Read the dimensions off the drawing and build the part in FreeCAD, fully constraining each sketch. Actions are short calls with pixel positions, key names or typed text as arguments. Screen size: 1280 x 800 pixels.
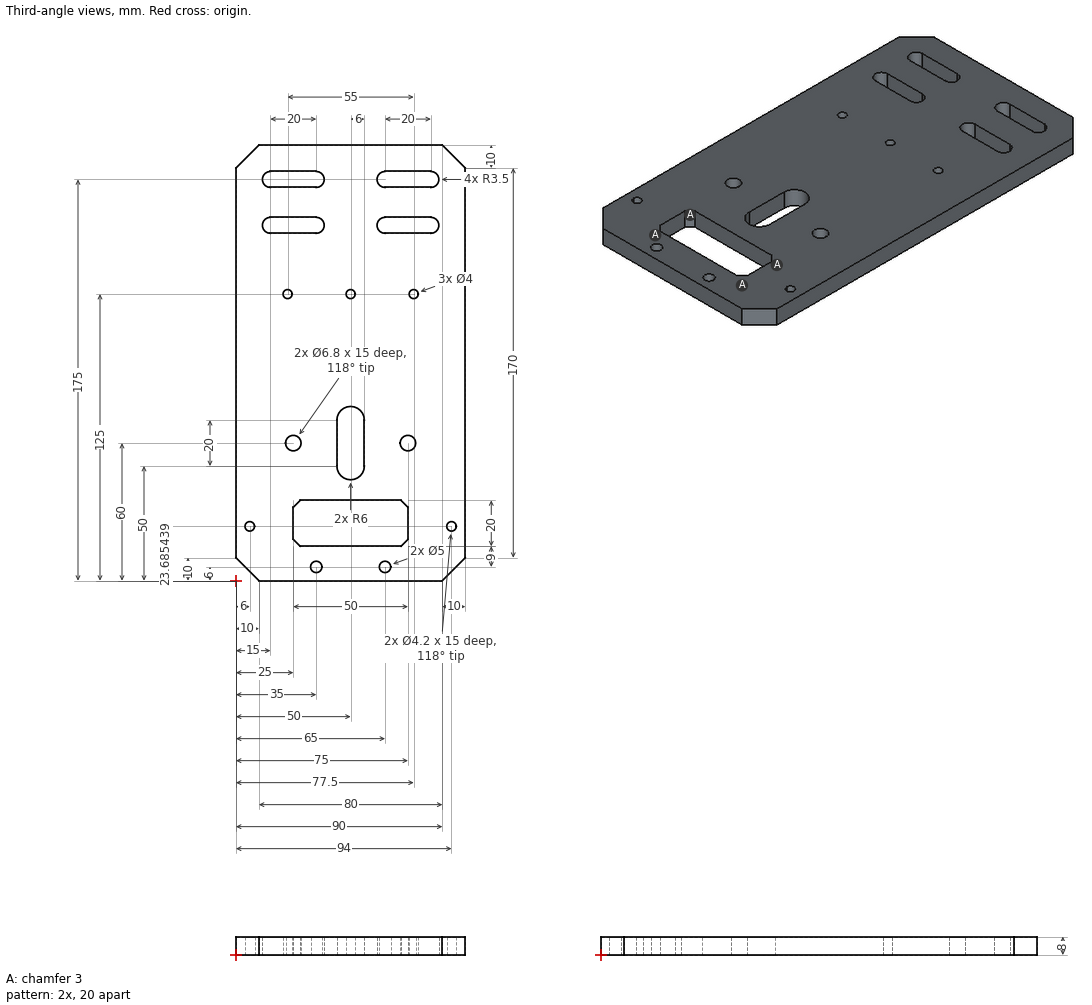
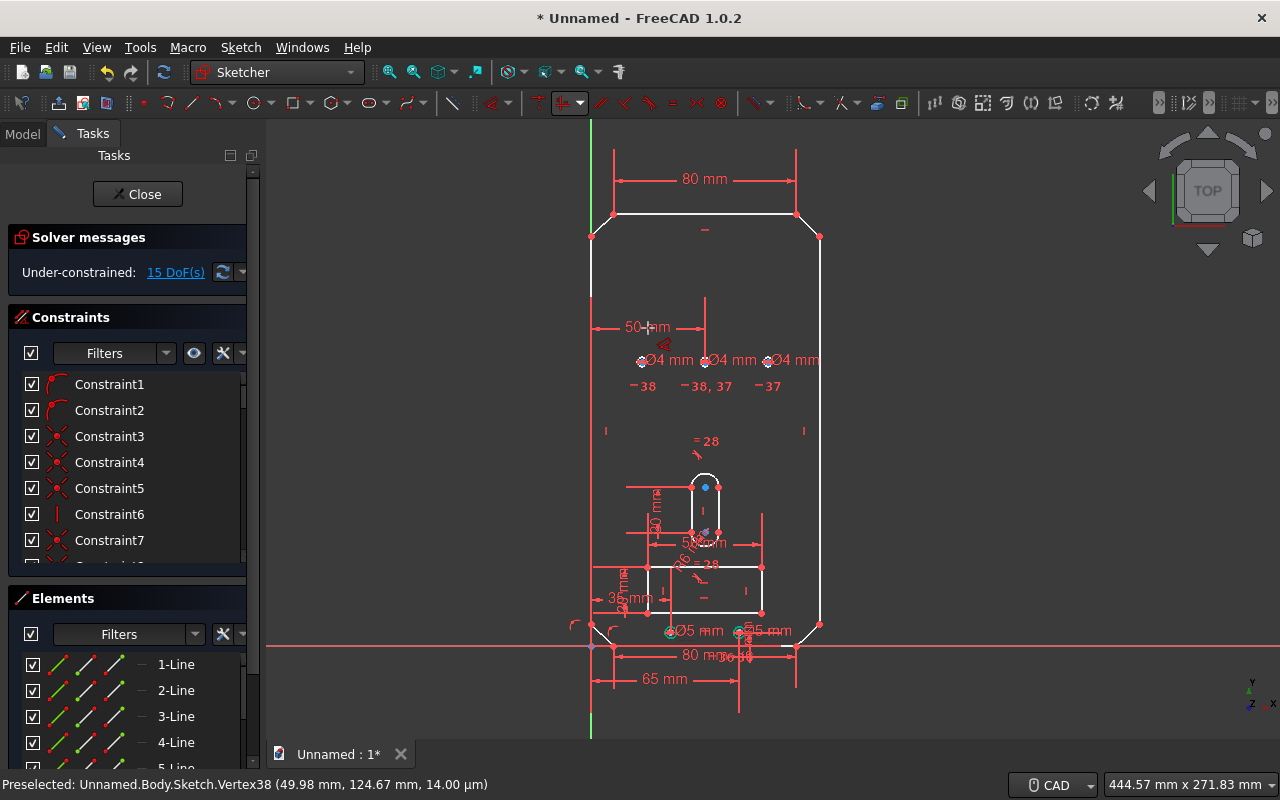
scroll(762, 613, up, 4)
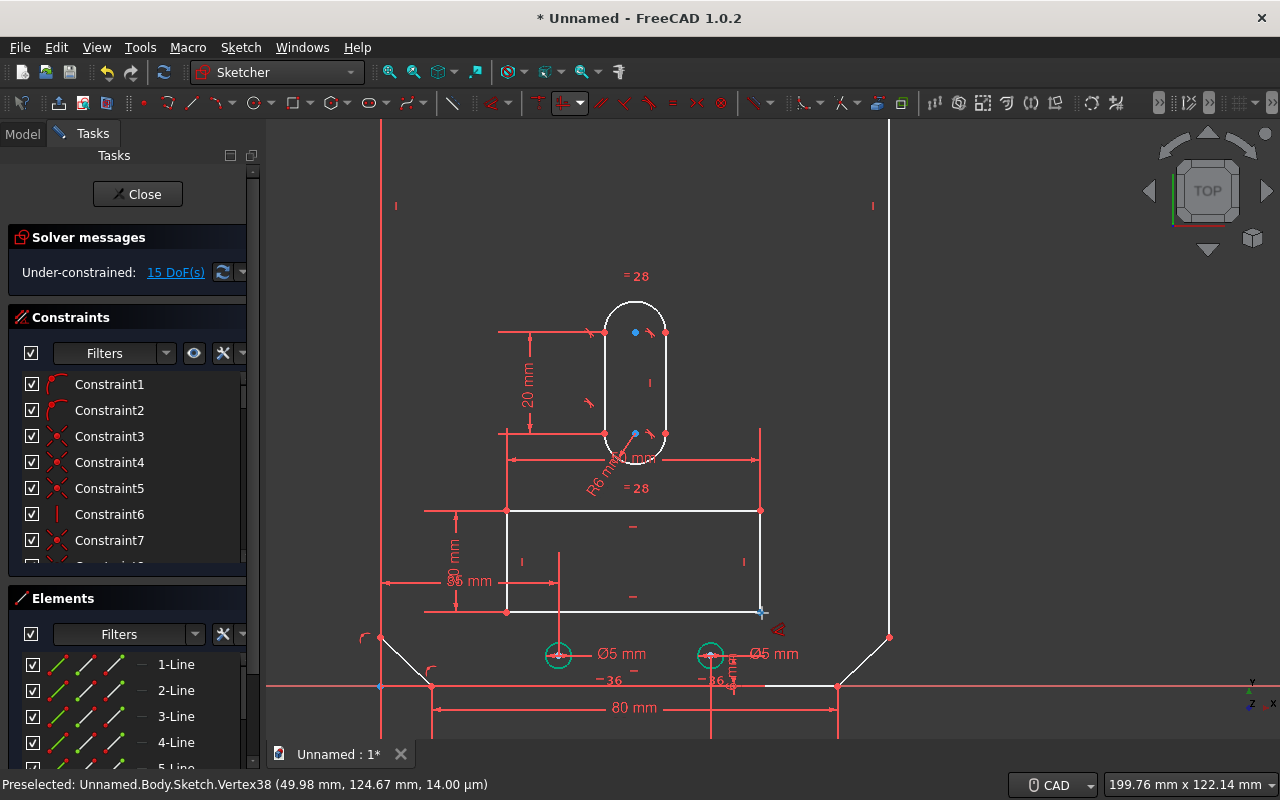
click(760, 612)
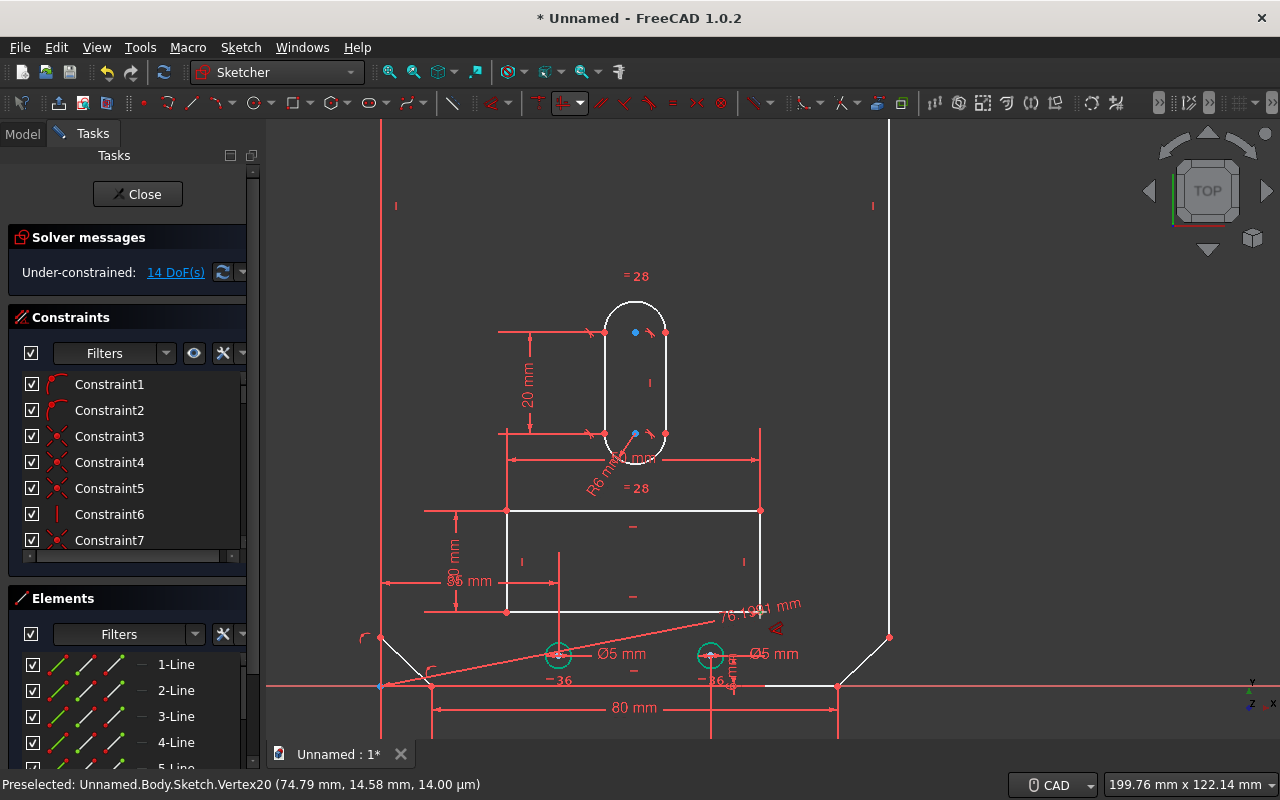
click(711, 656)
click(794, 634)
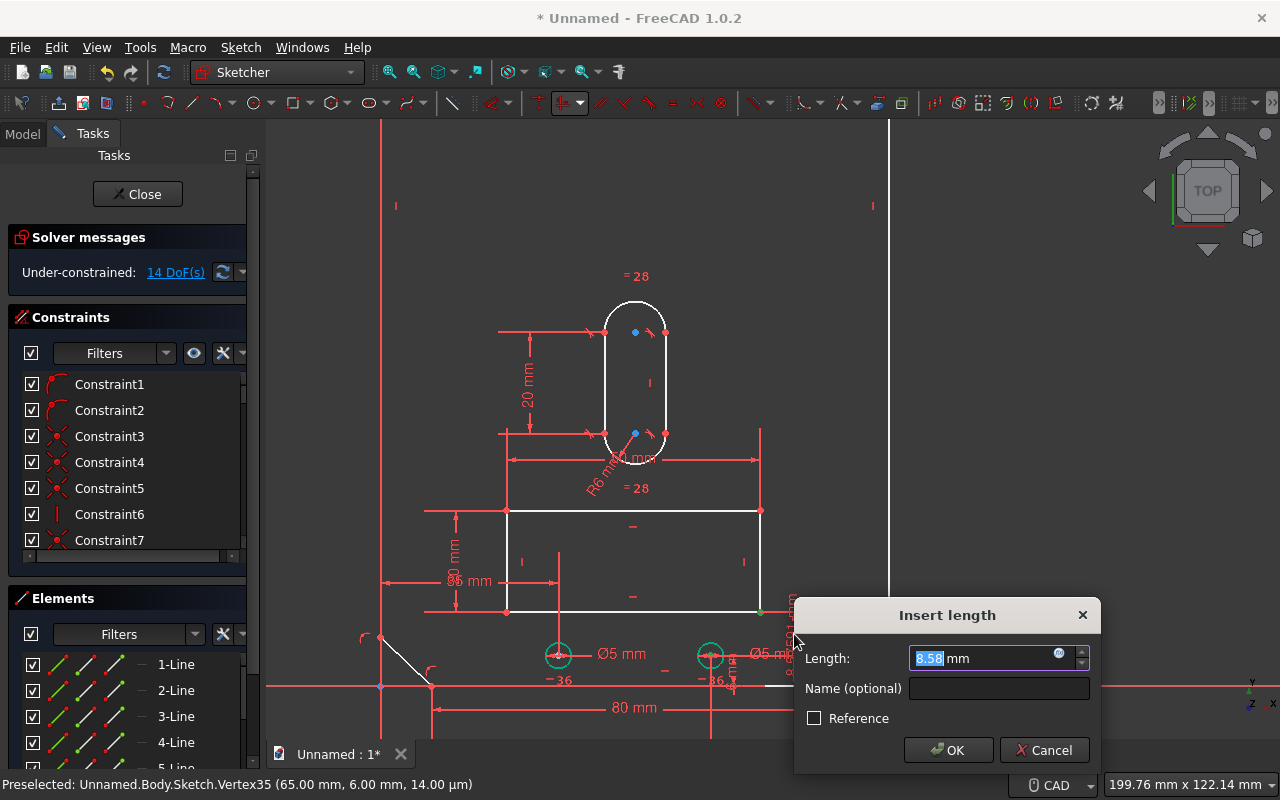
text(9)
key(Return)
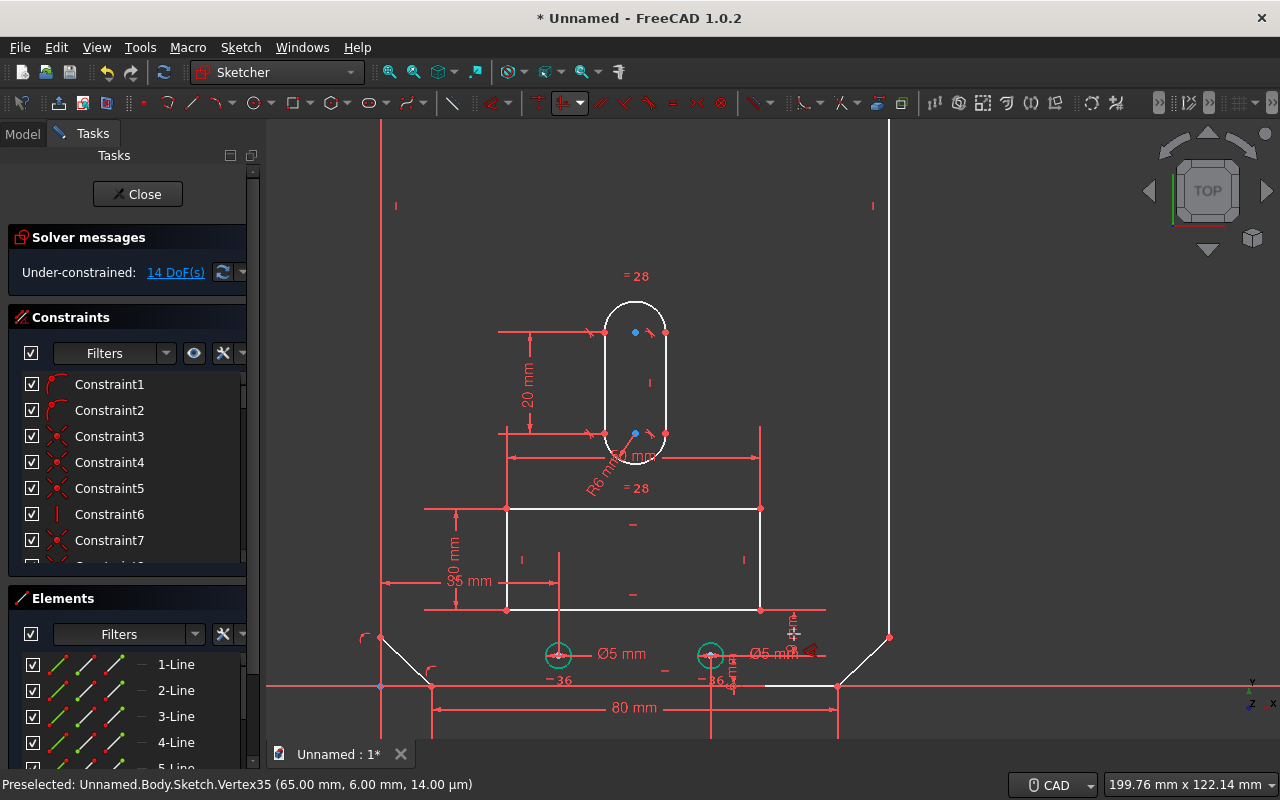
scroll(666, 332, up, 2)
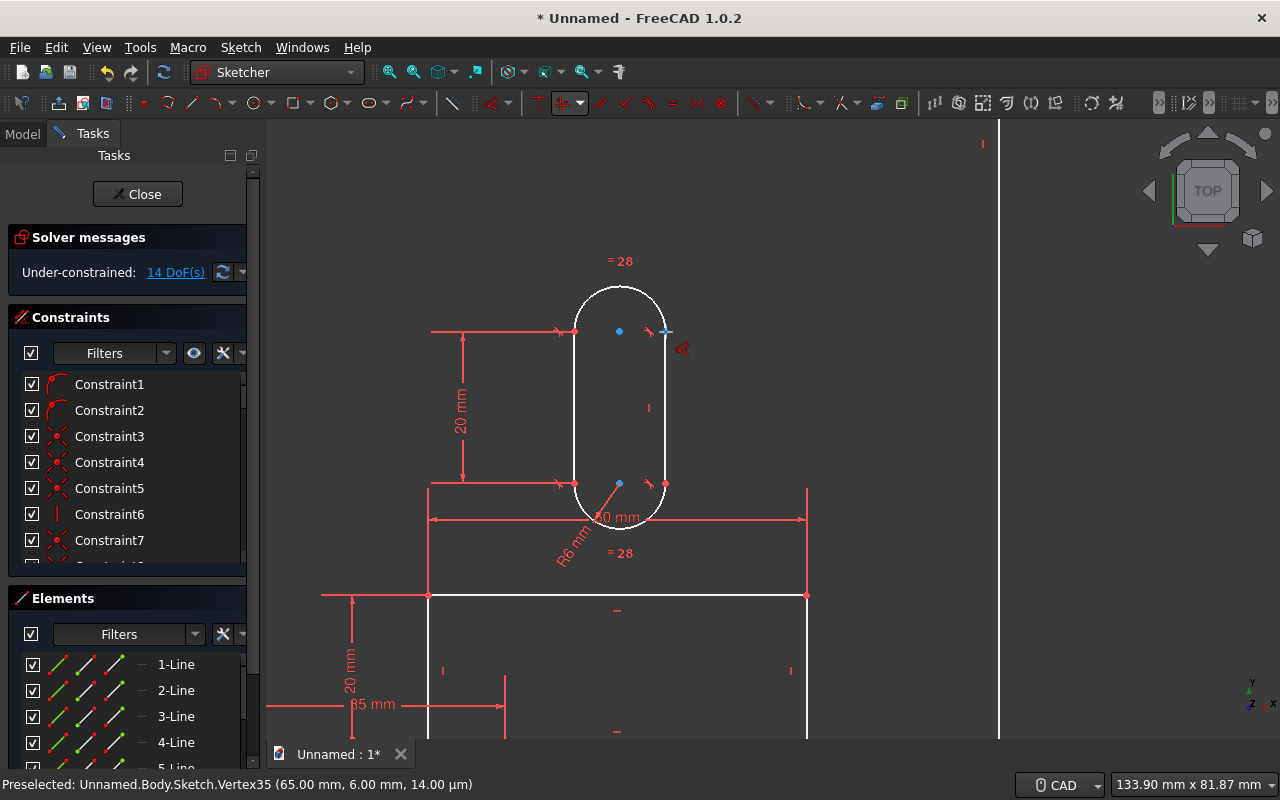
click(665, 332)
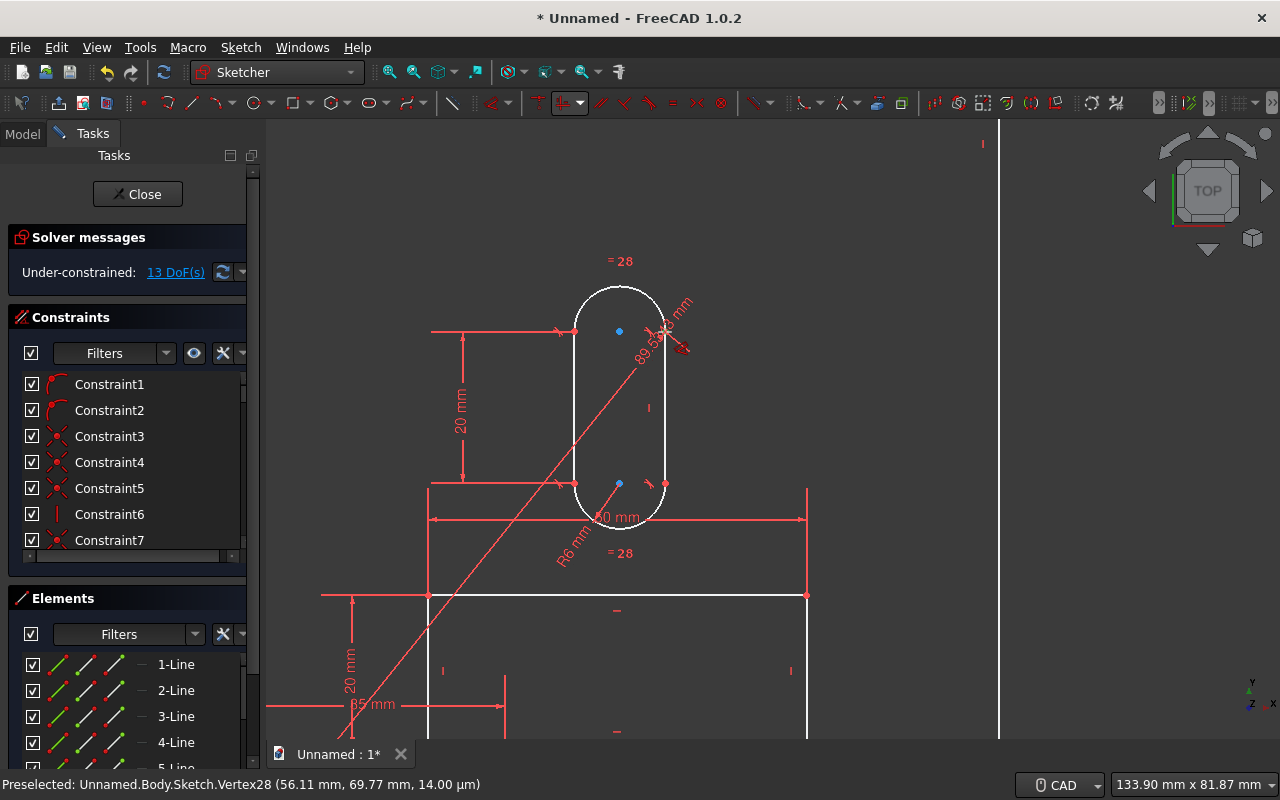
scroll(741, 553, down, 6)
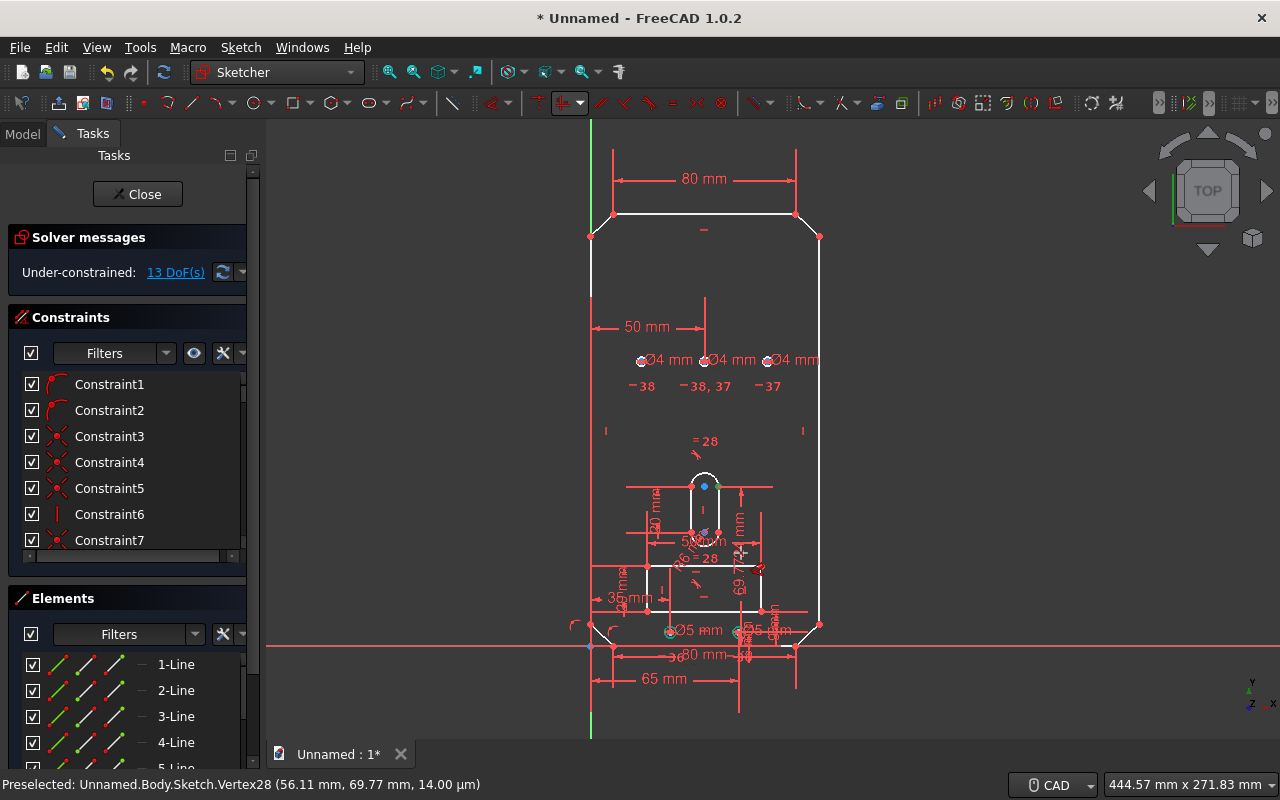
scroll(705, 362, up, 6)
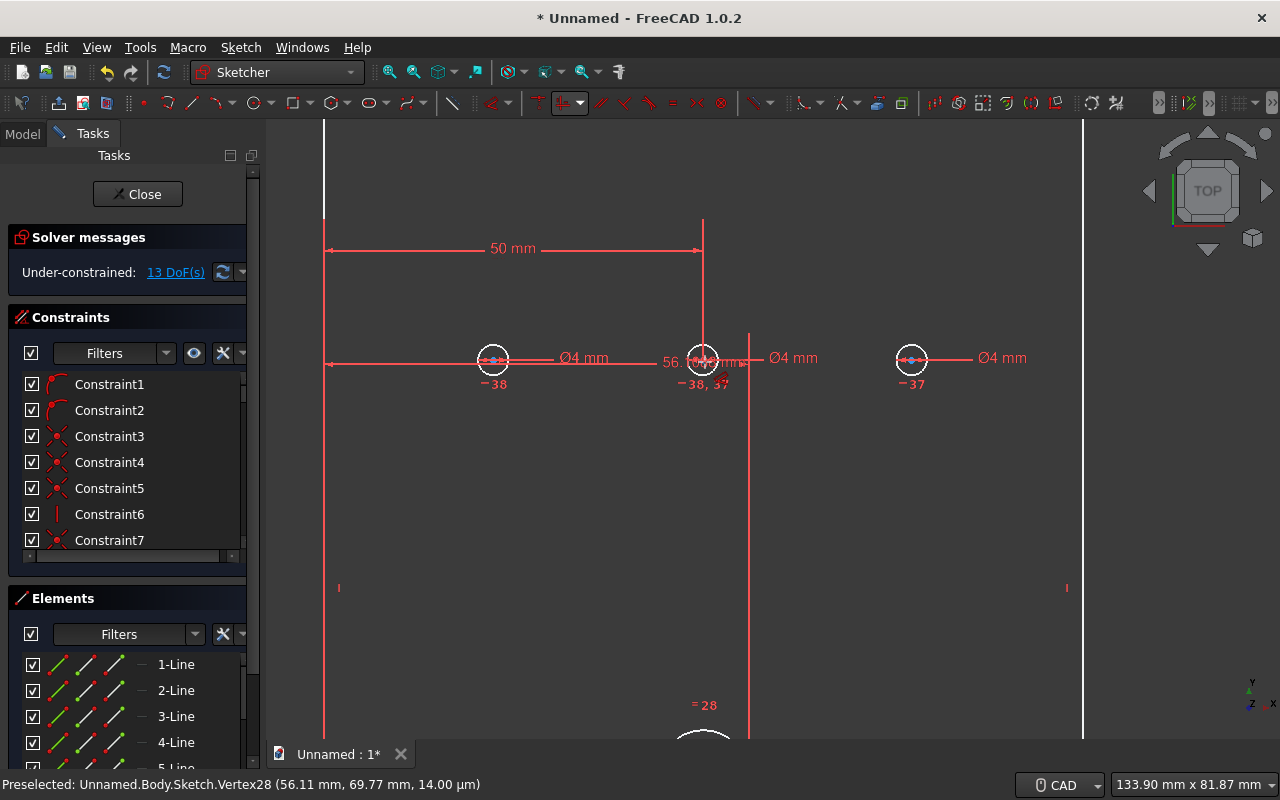
click(703, 360)
click(726, 326)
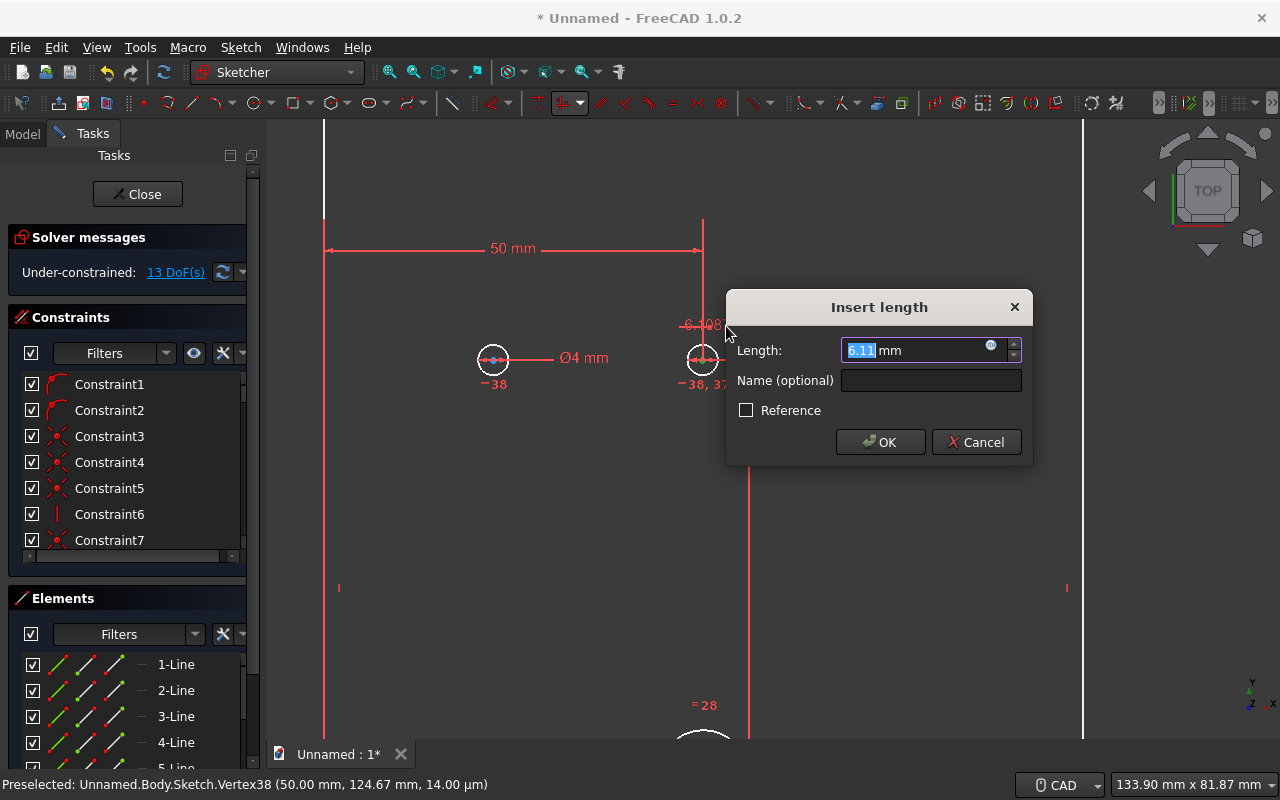
text(6)
key(Return)